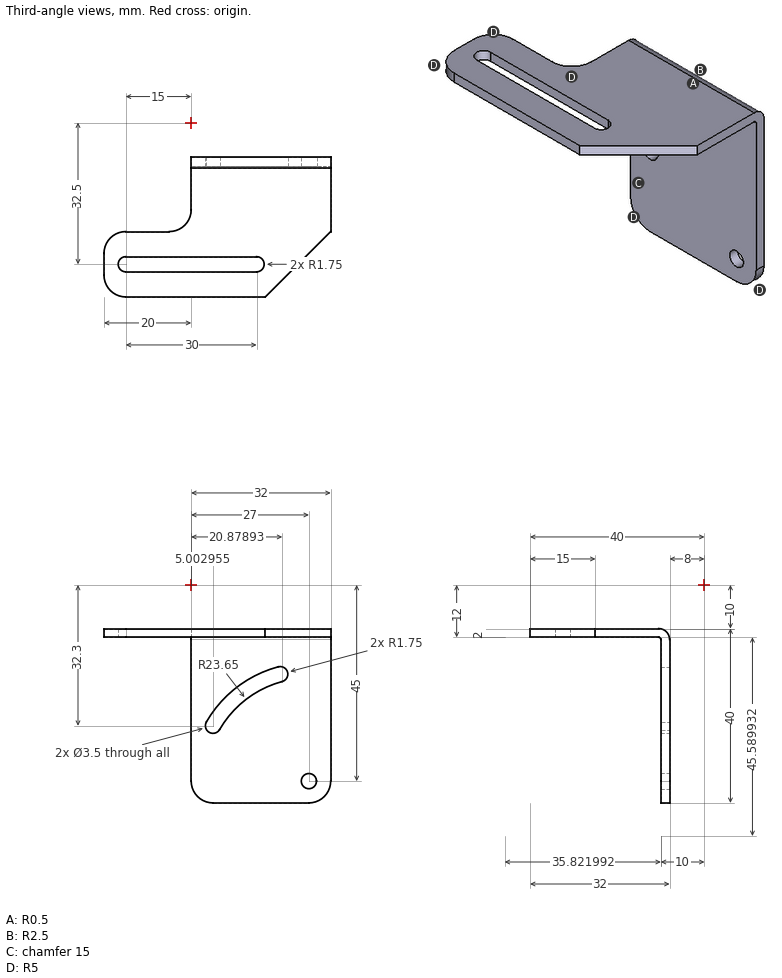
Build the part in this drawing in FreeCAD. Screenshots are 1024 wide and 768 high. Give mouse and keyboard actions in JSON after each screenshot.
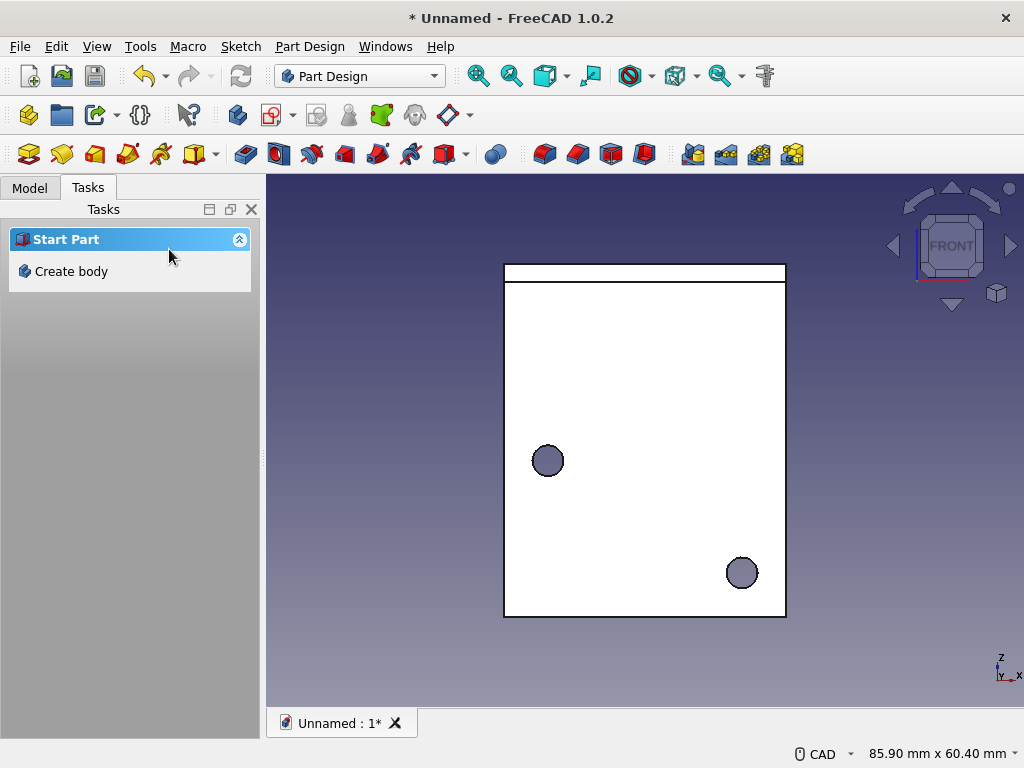
{"action": "key", "text": "3"}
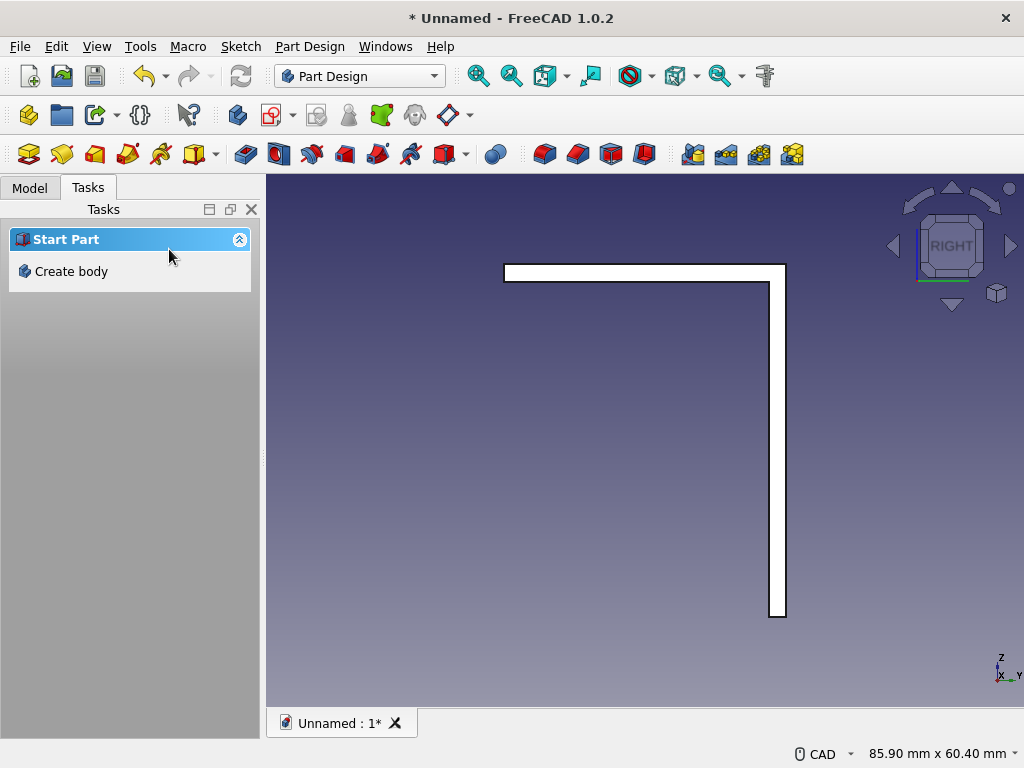
{"action": "key", "text": "5"}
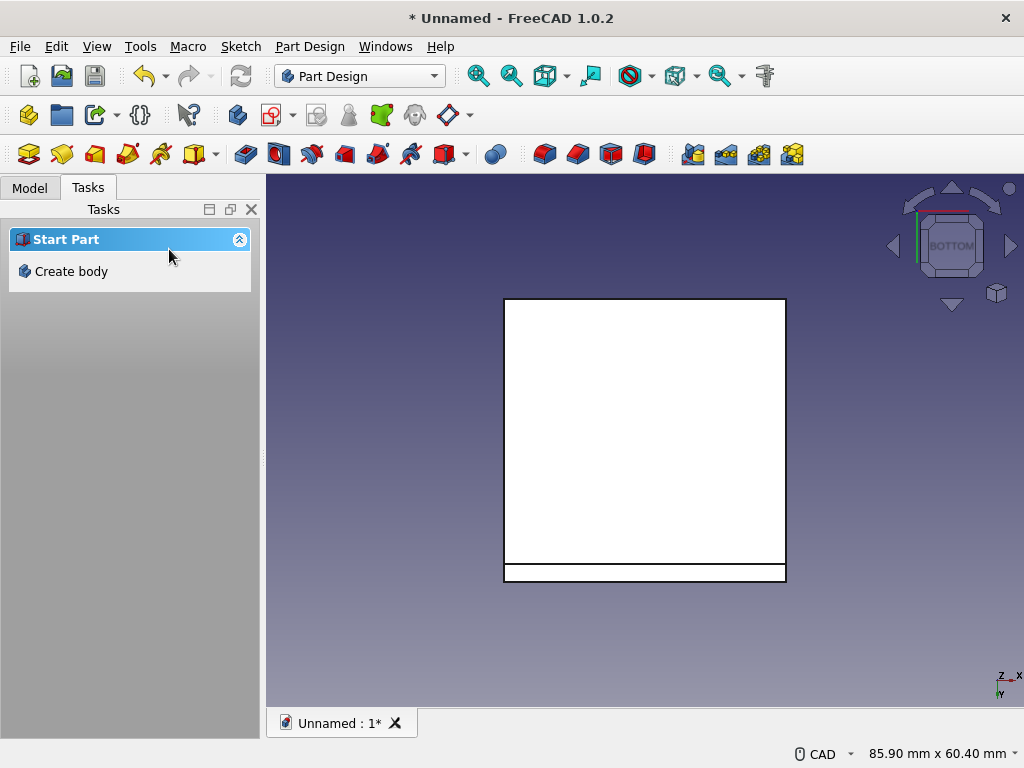
{"action": "key", "text": "4"}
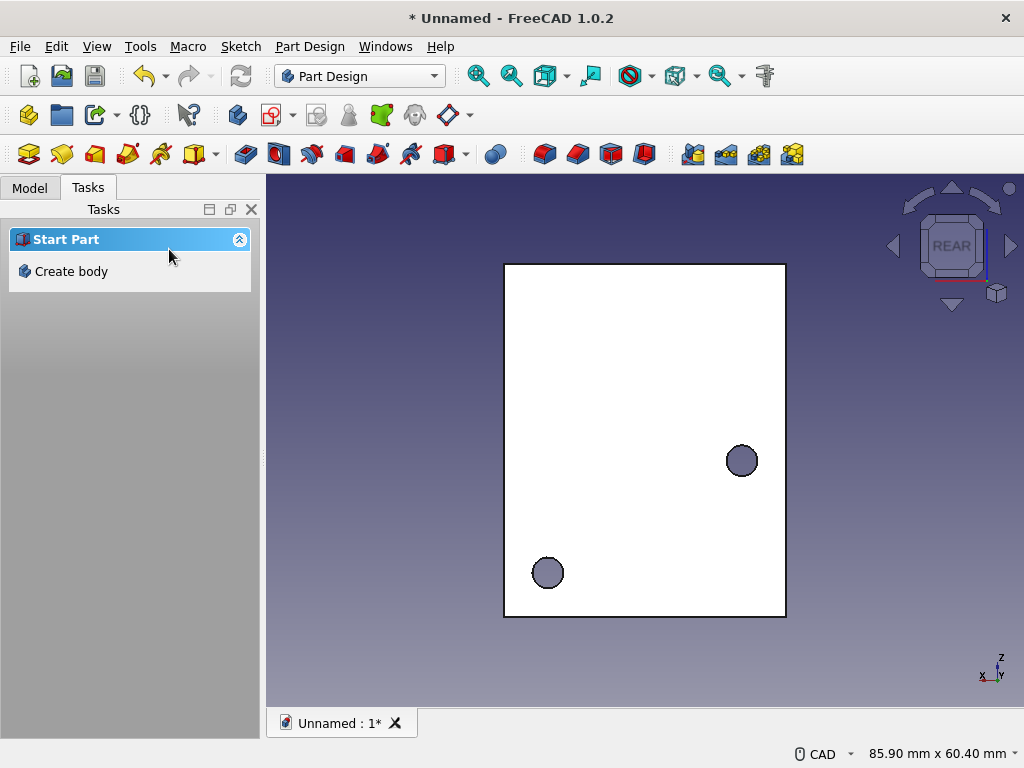
{"action": "key", "text": "6"}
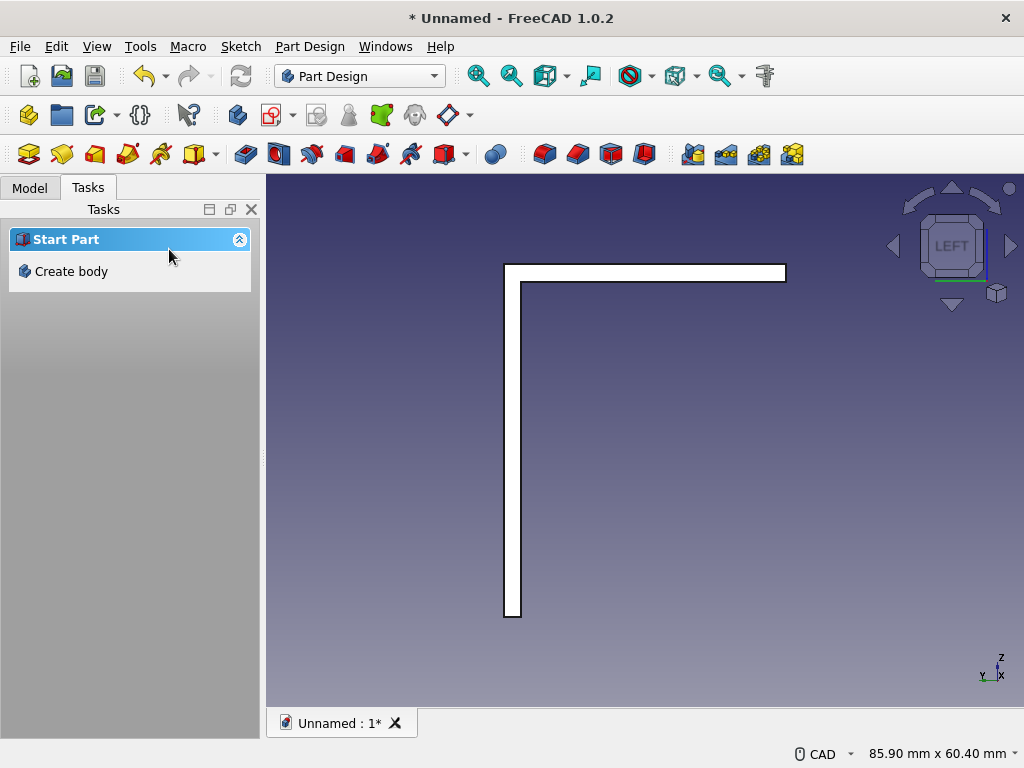
{"action": "key", "text": "v 3"}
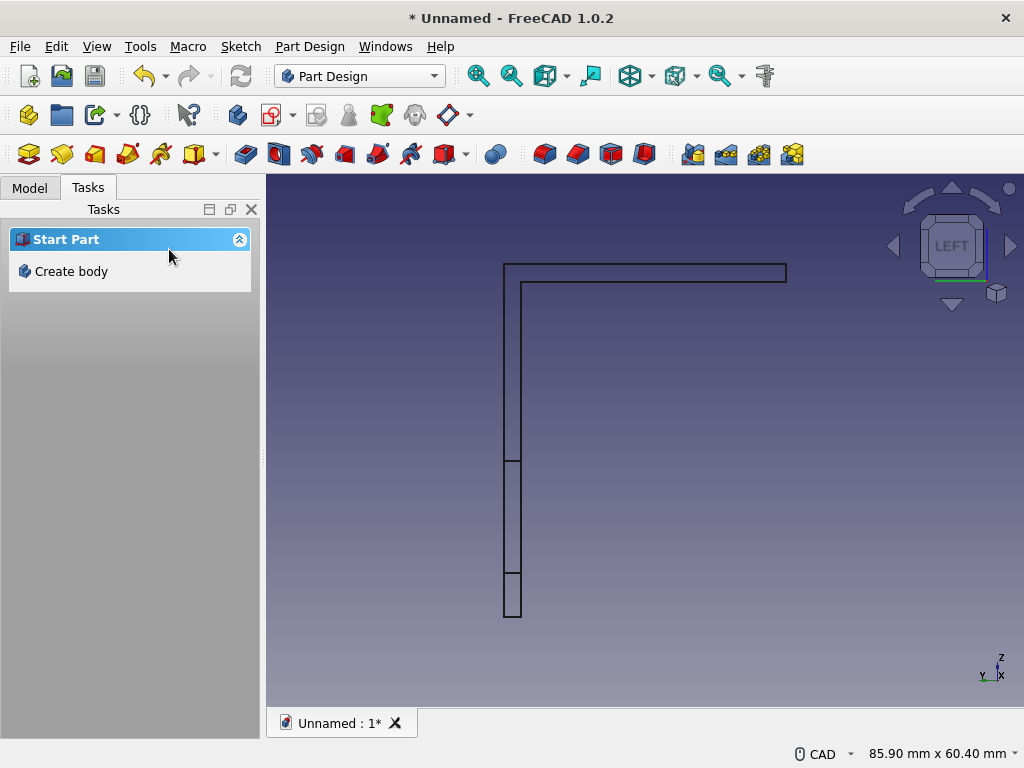
{"action": "key", "text": "0"}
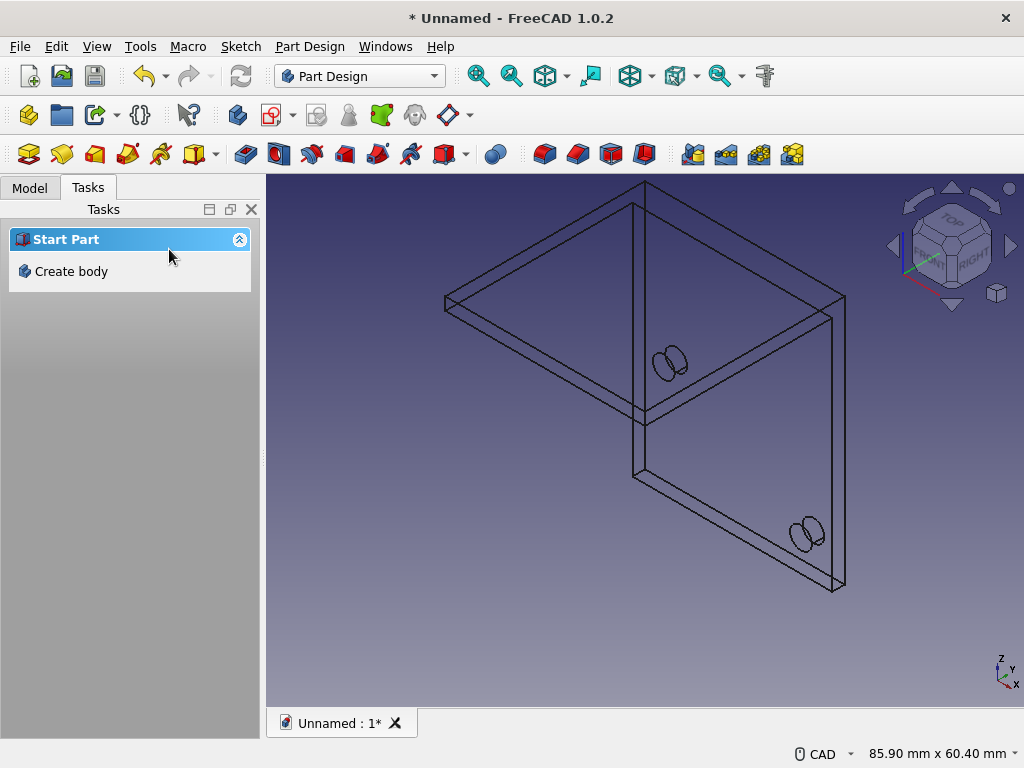
{"action": "left_click", "coordinate": [732, 259]}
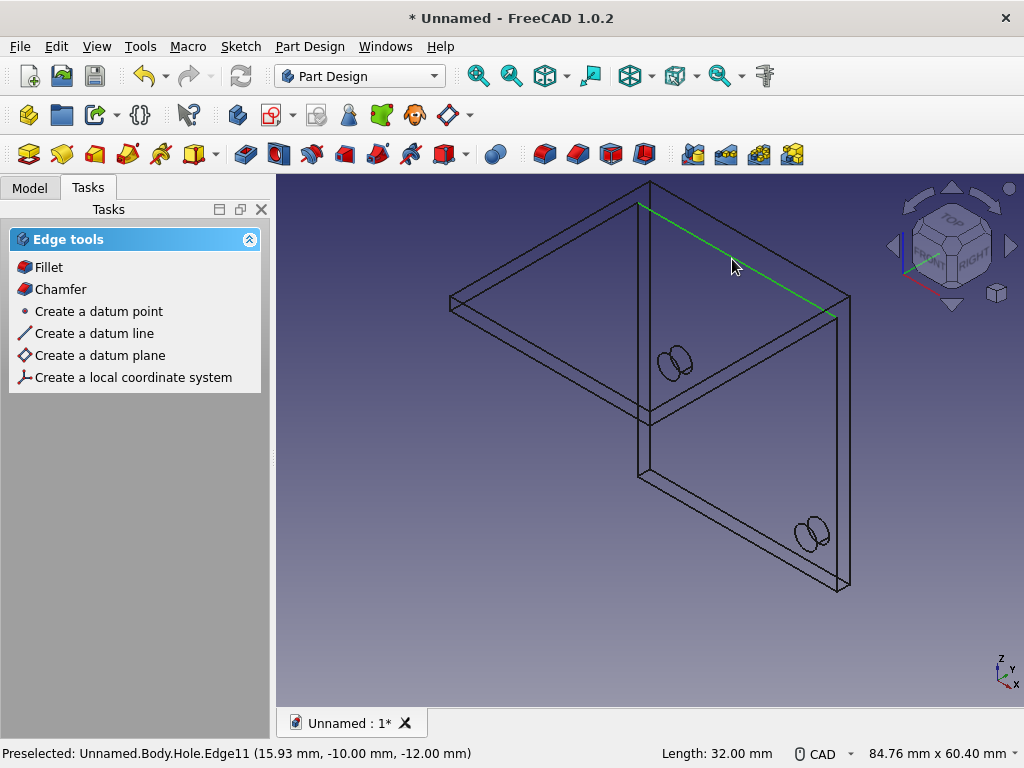
{"action": "key", "text": "v 1"}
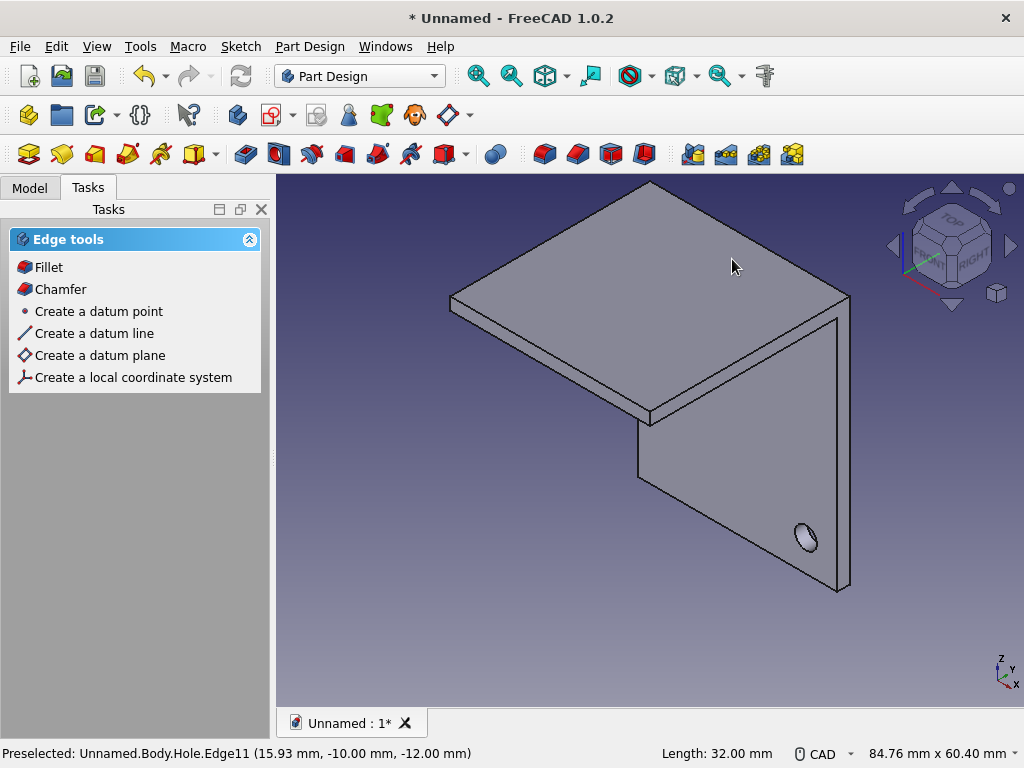
{"action": "left_click", "coordinate": [545, 154]}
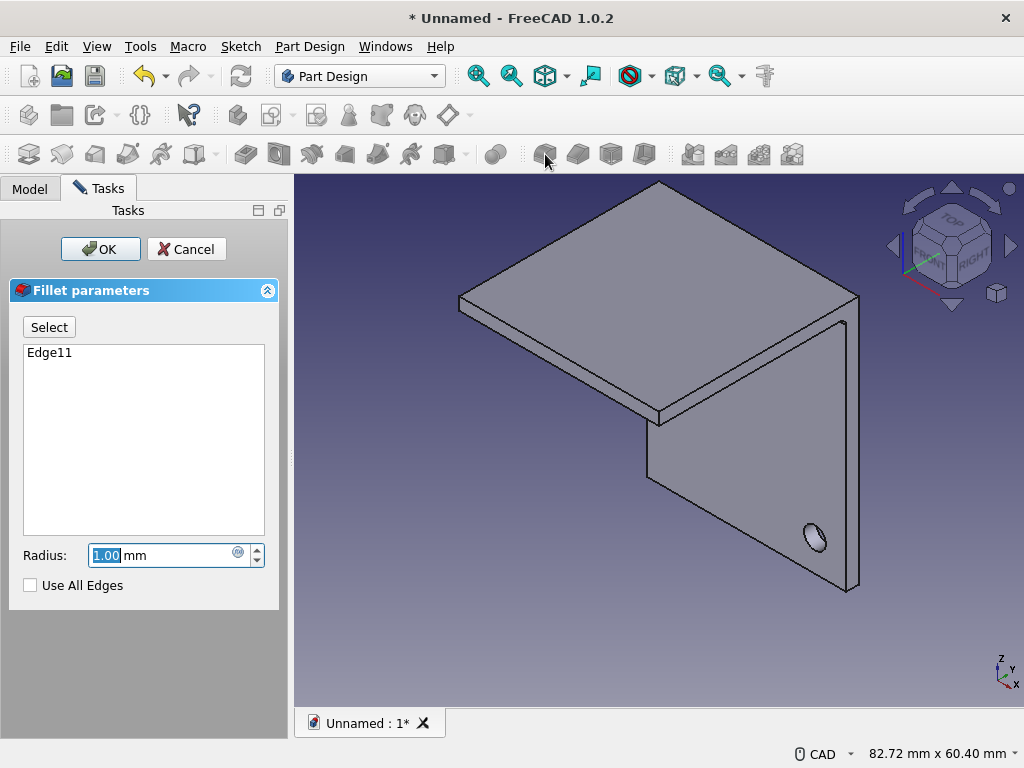
{"action": "type", "text": "0.5"}
{"action": "key", "text": "Tab"}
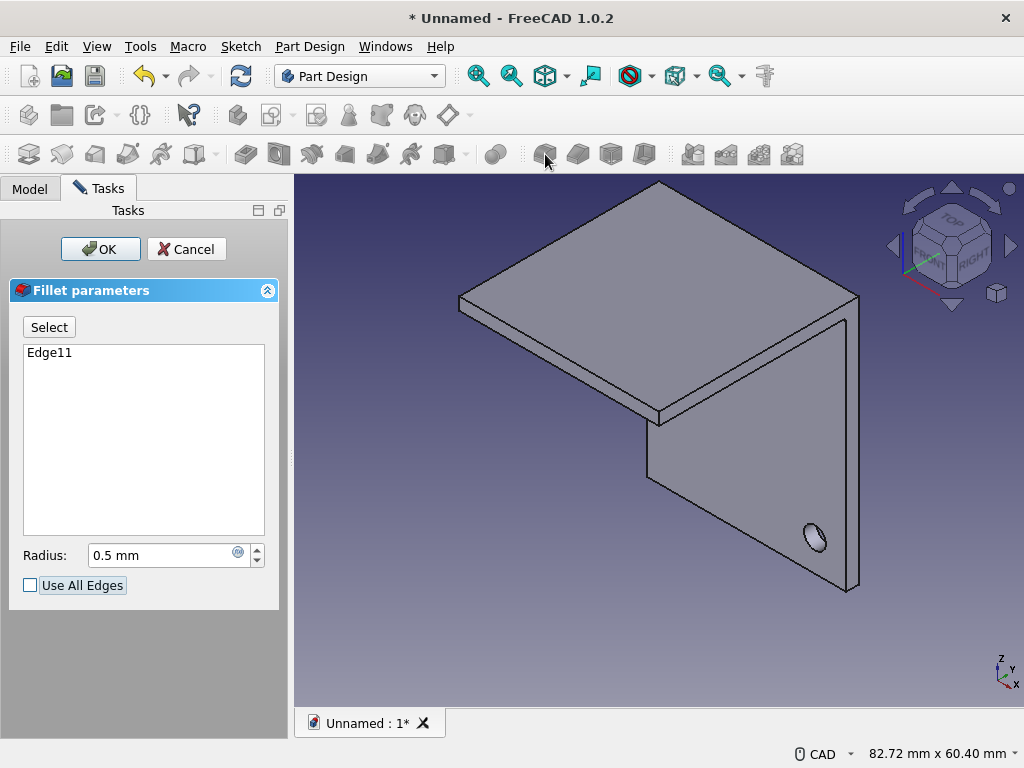
{"action": "left_click", "coordinate": [101, 249]}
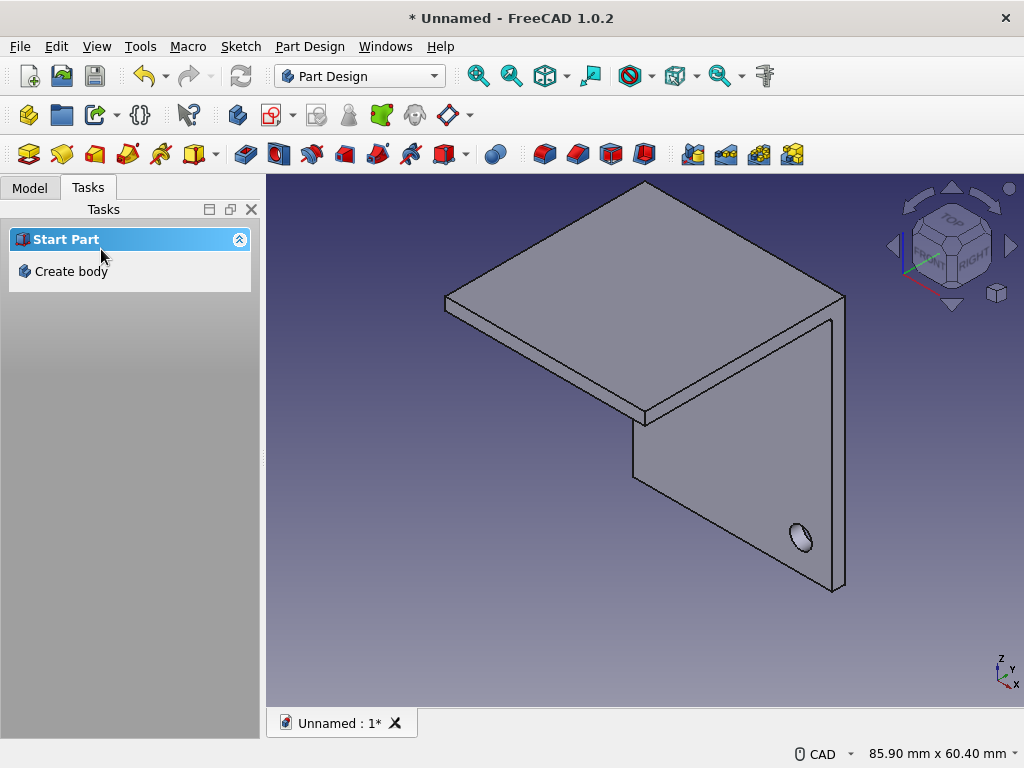
{"action": "key", "text": "2"}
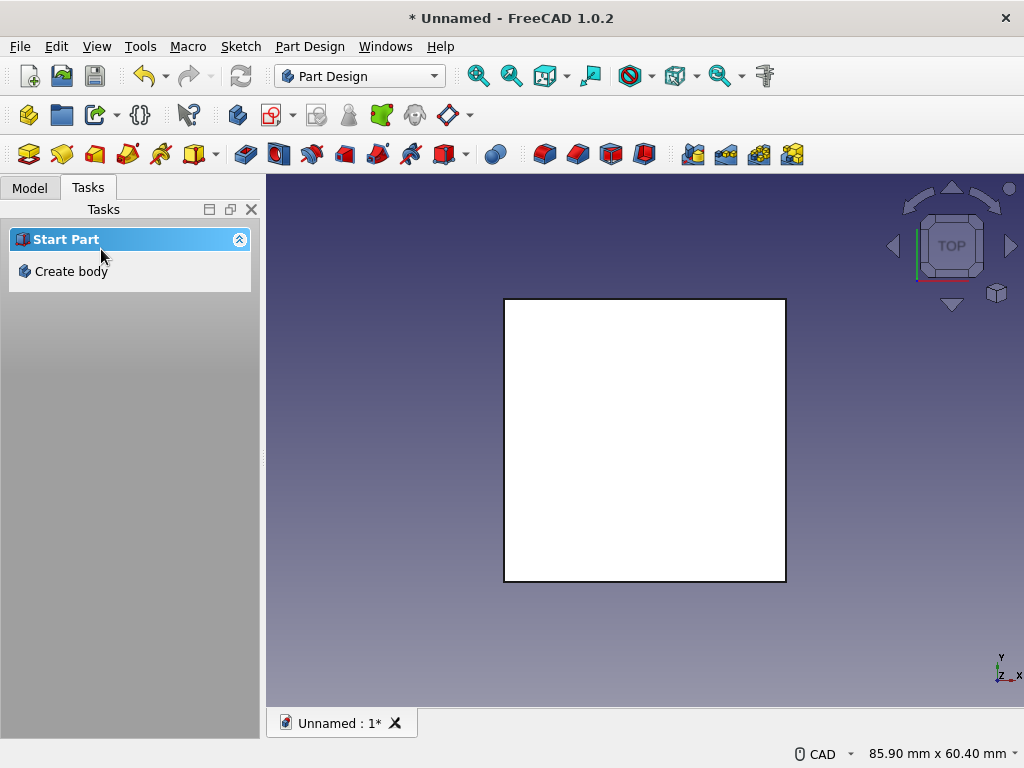
{"action": "left_click", "coordinate": [645, 298]}